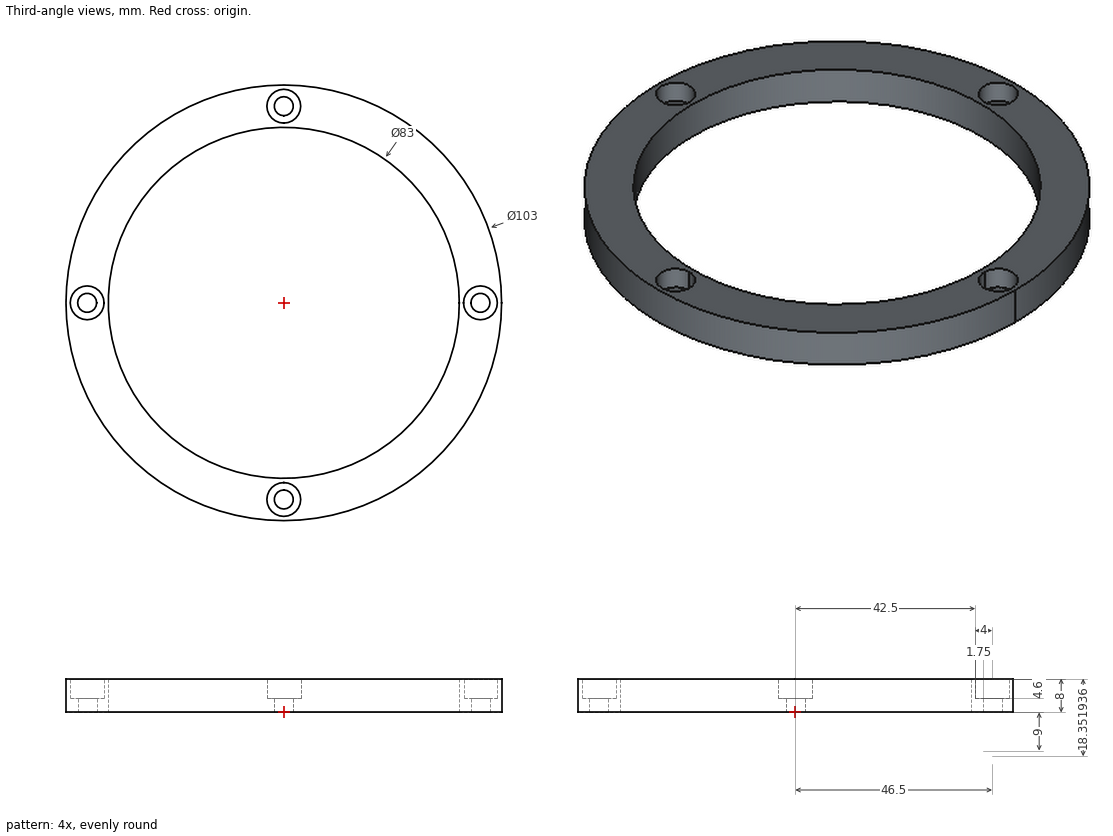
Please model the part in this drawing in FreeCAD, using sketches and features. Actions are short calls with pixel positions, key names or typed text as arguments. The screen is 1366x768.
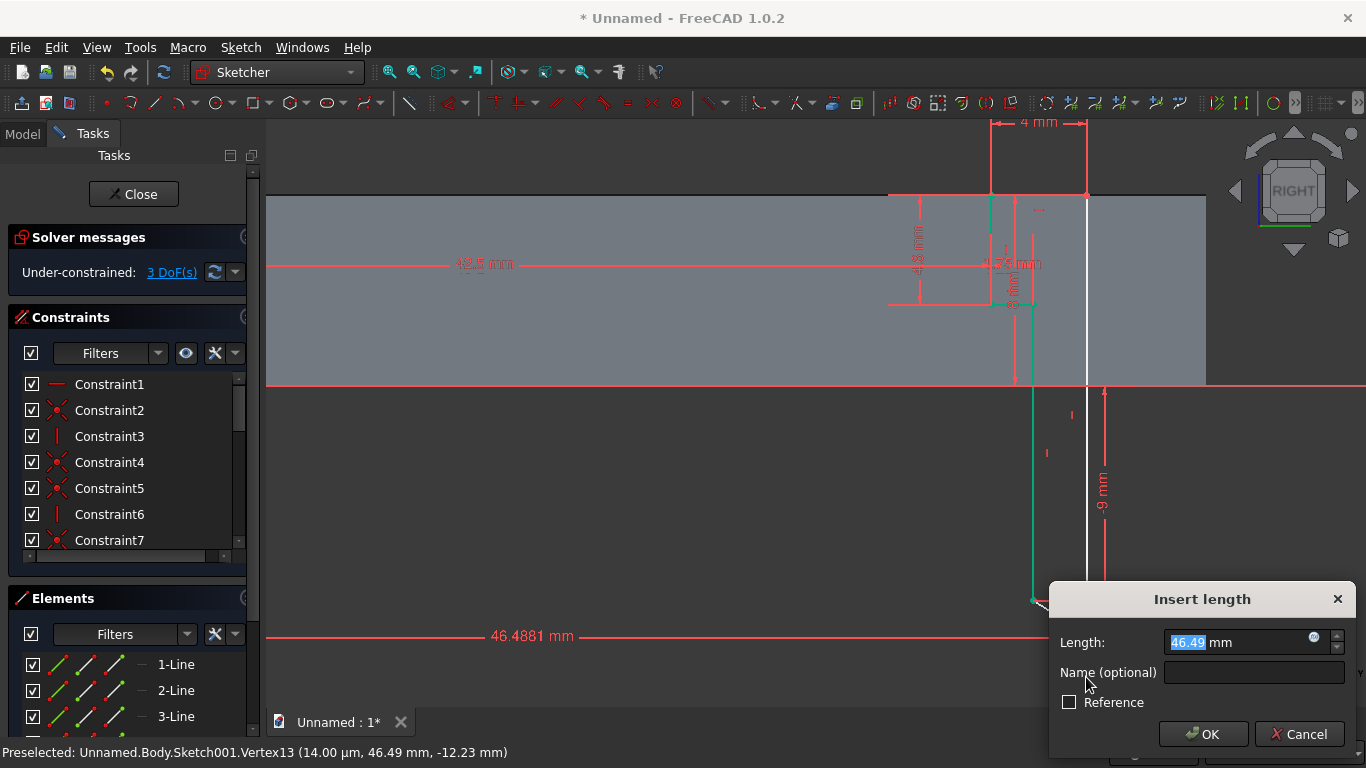
text(46.5)
key(Return)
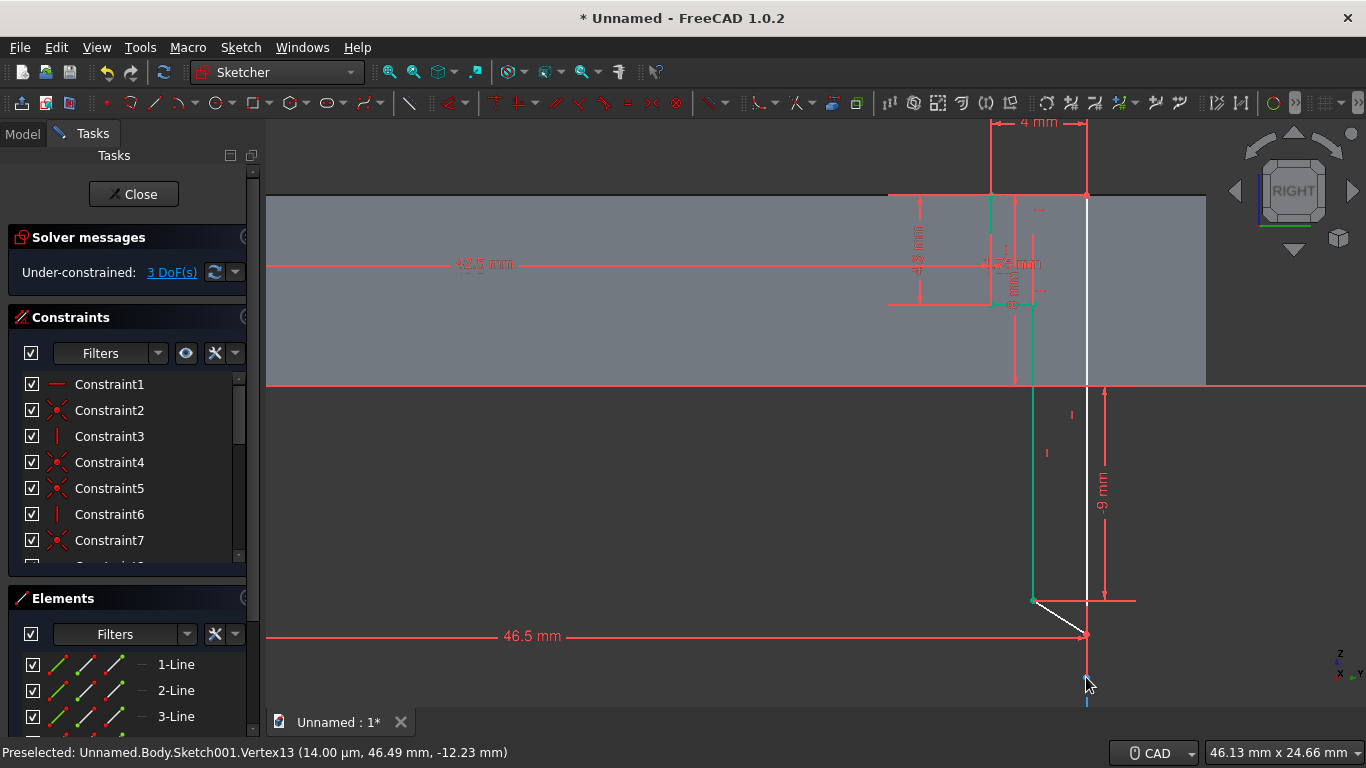
click(1087, 503)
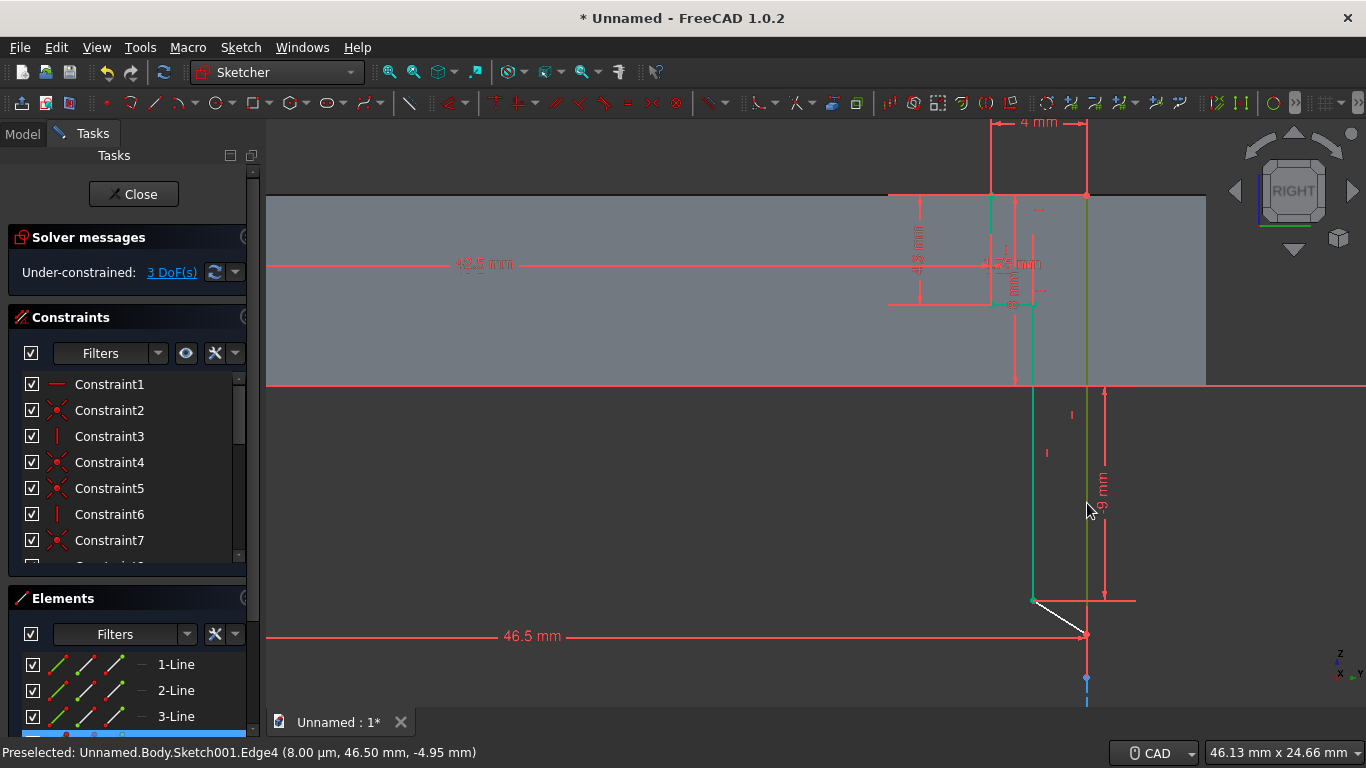
key(i)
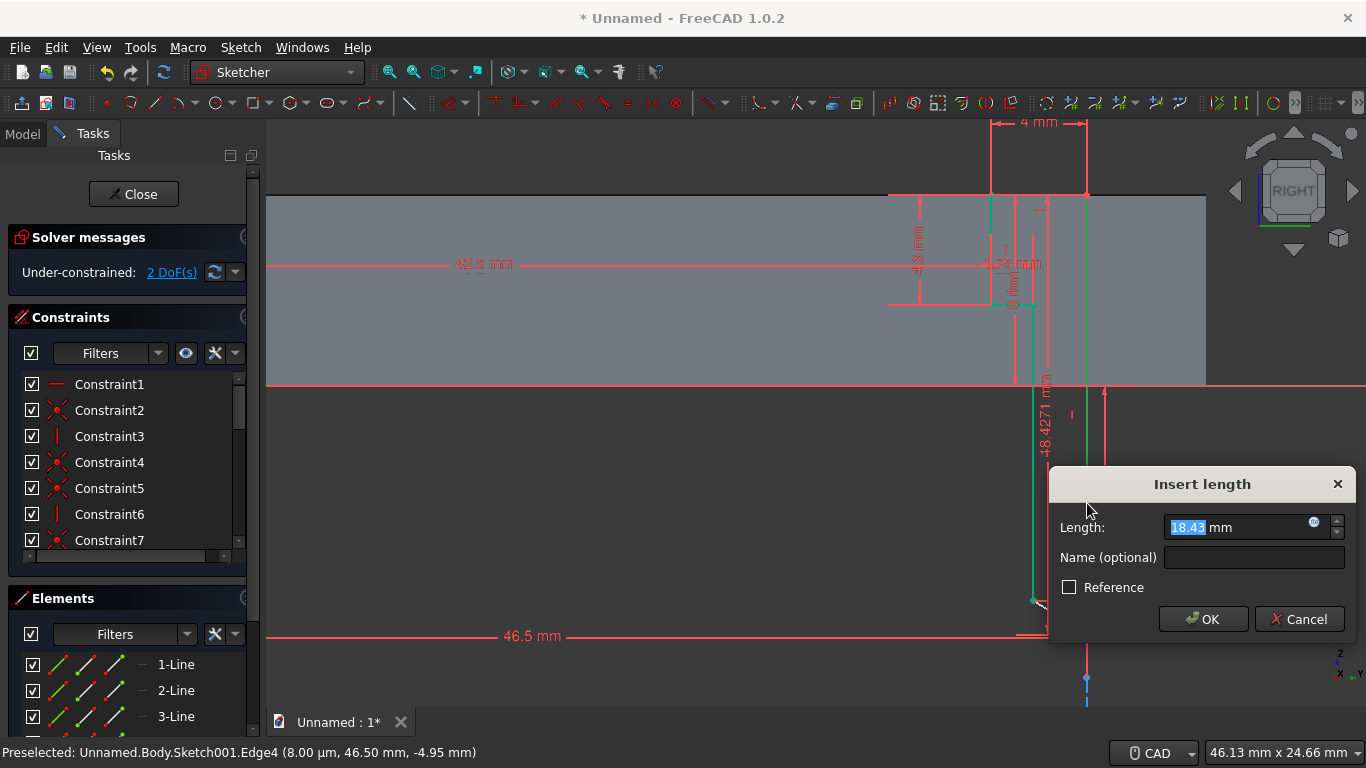
text(18.351936)
key(Return)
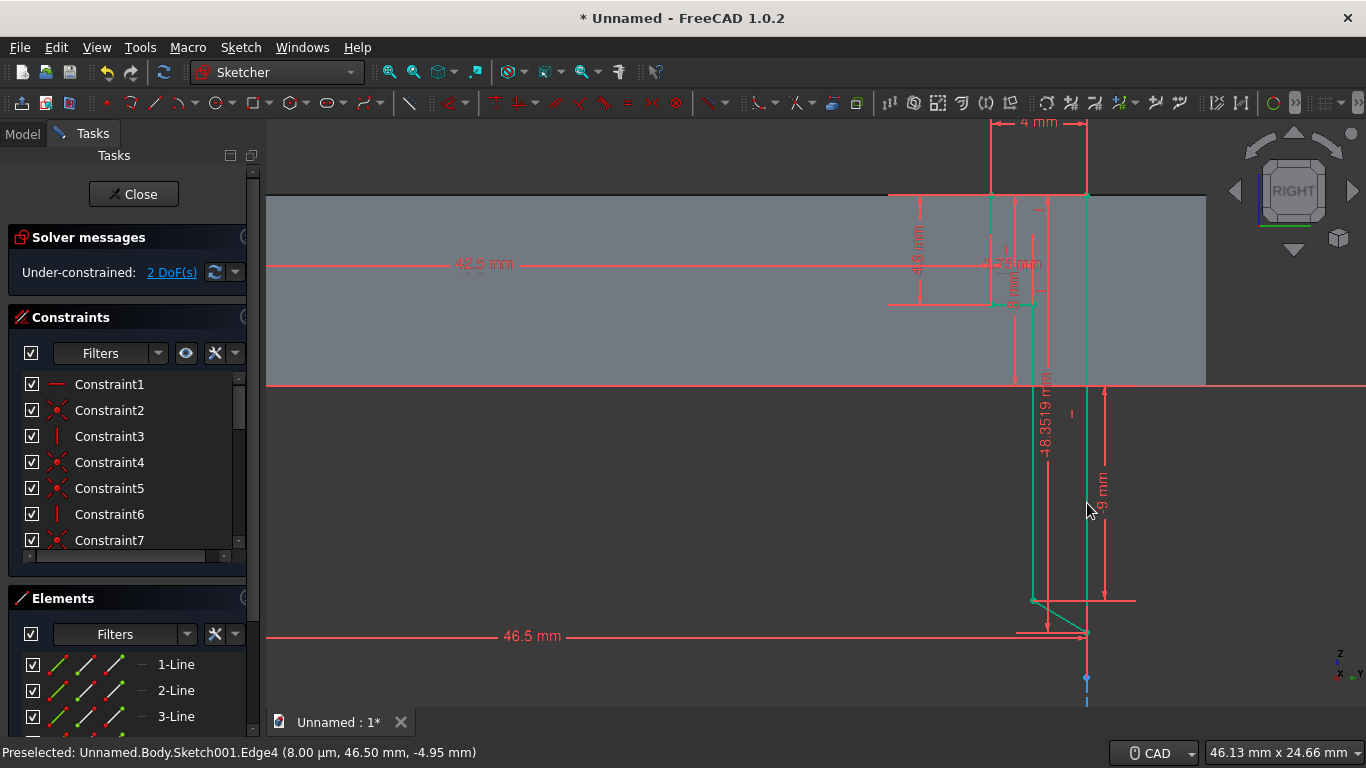
click(134, 194)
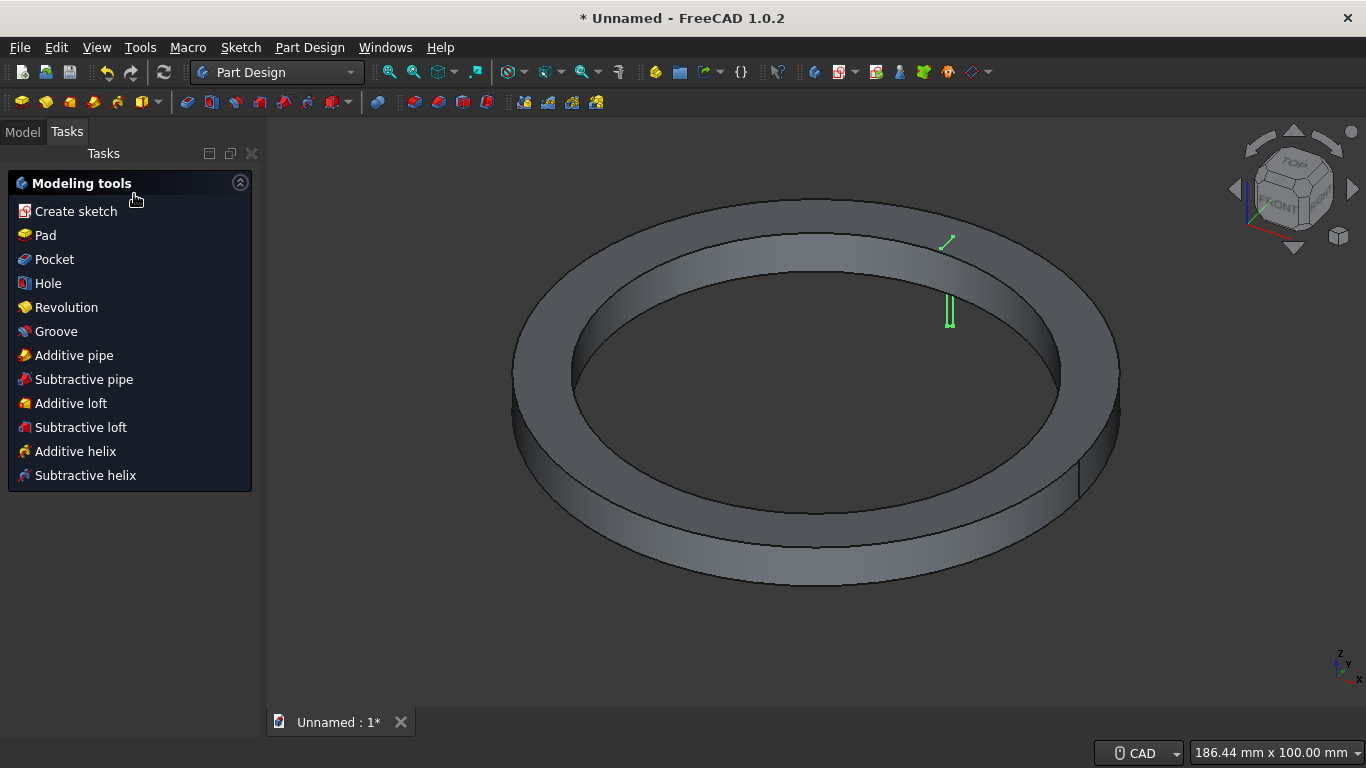
click(236, 102)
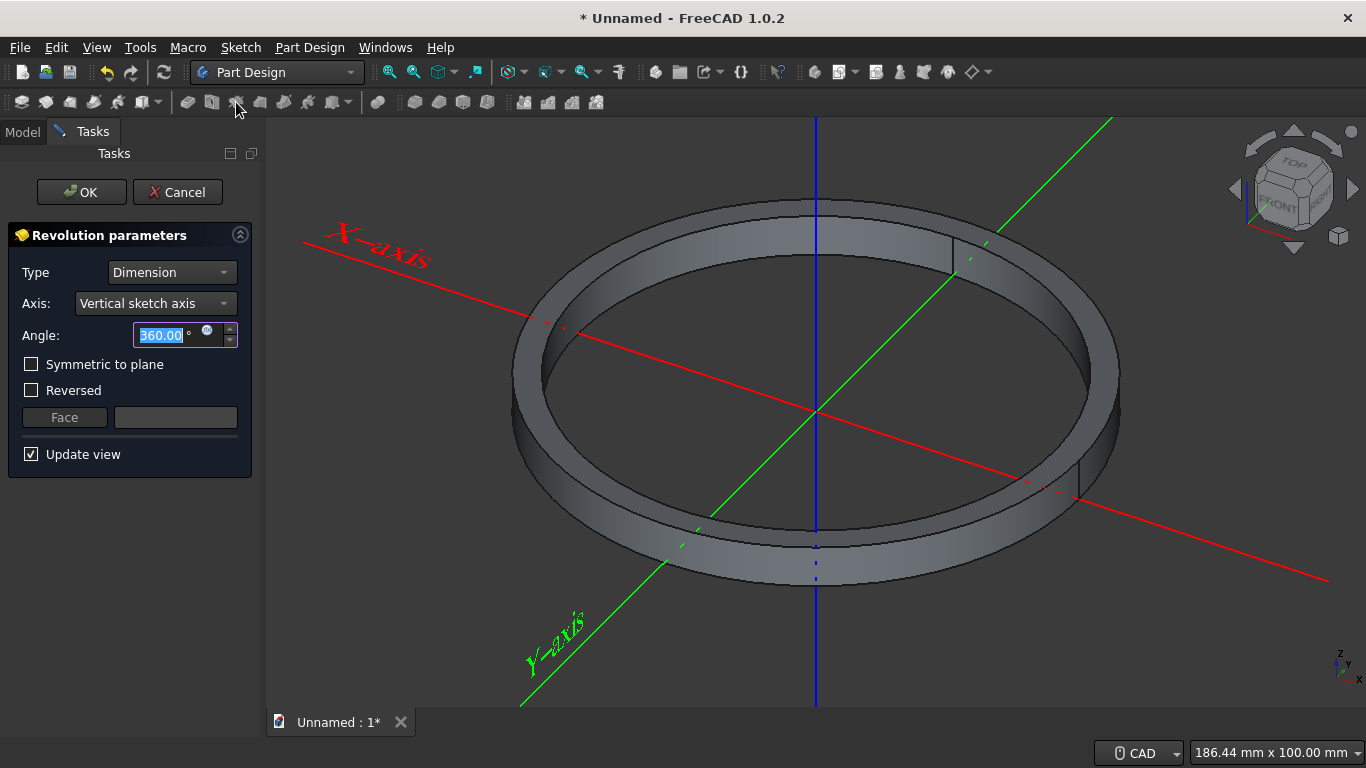
click(156, 304)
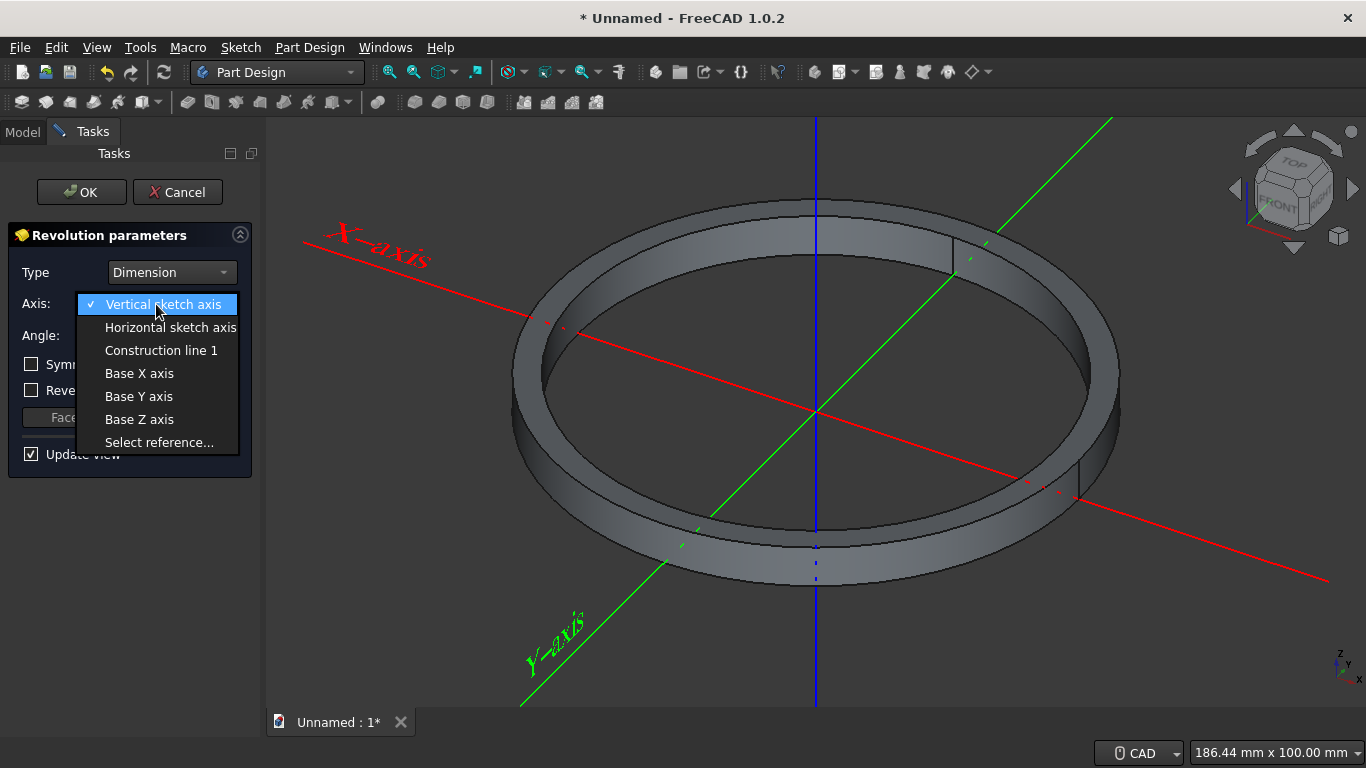
click(156, 350)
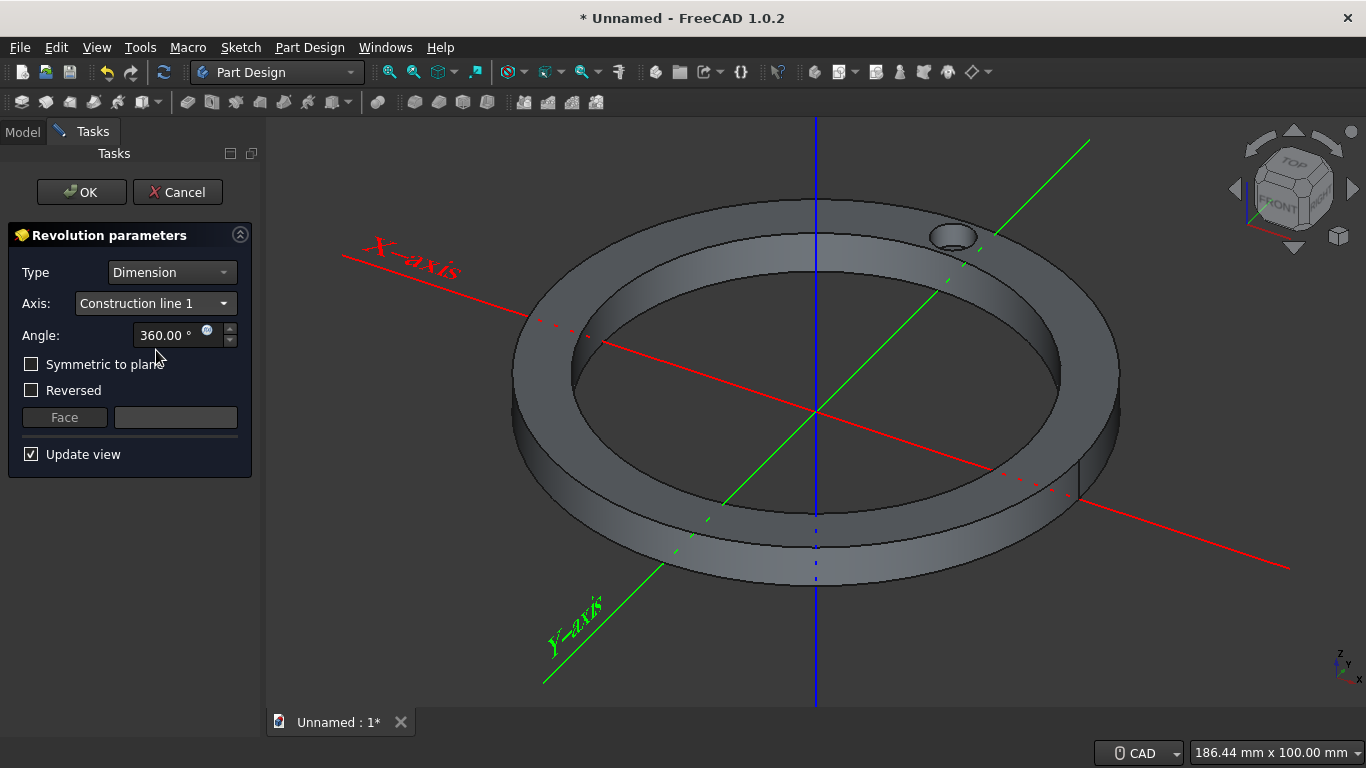
click(82, 192)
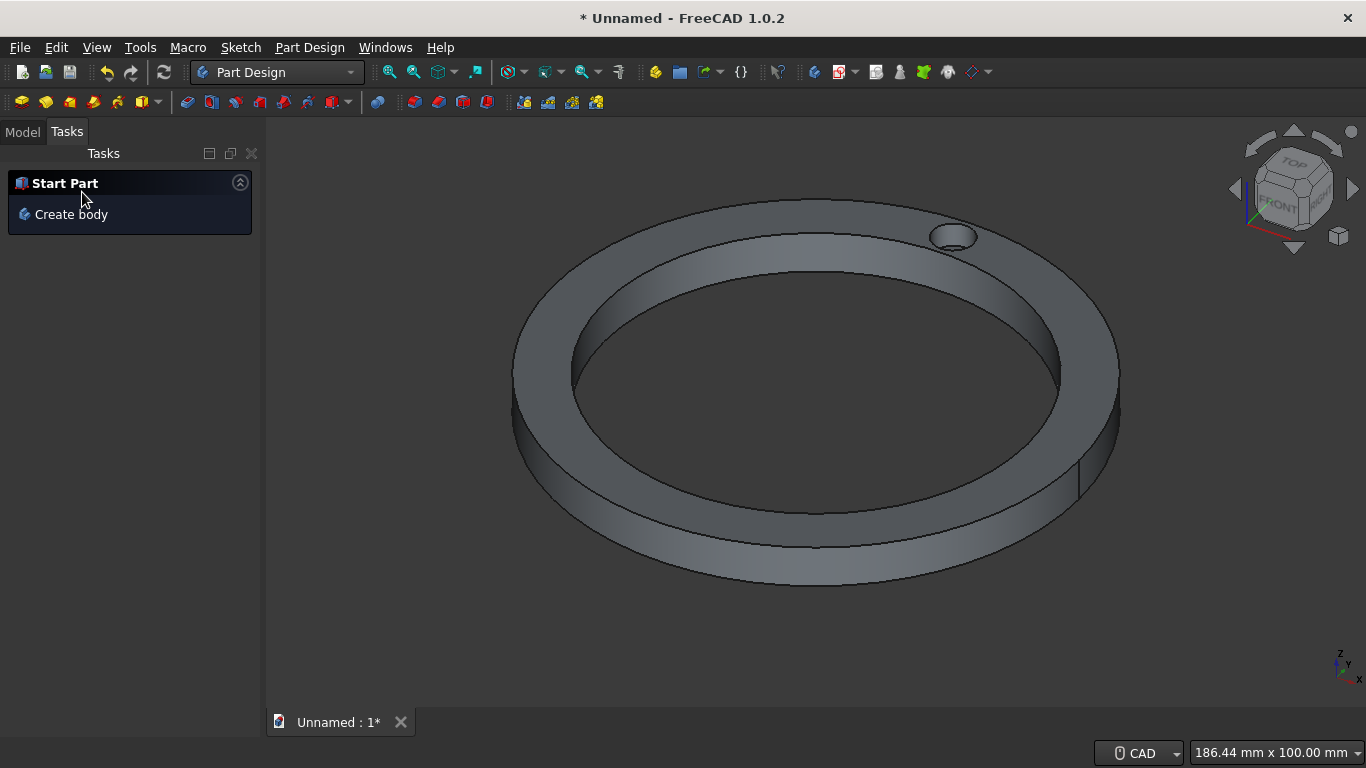
click(23, 131)